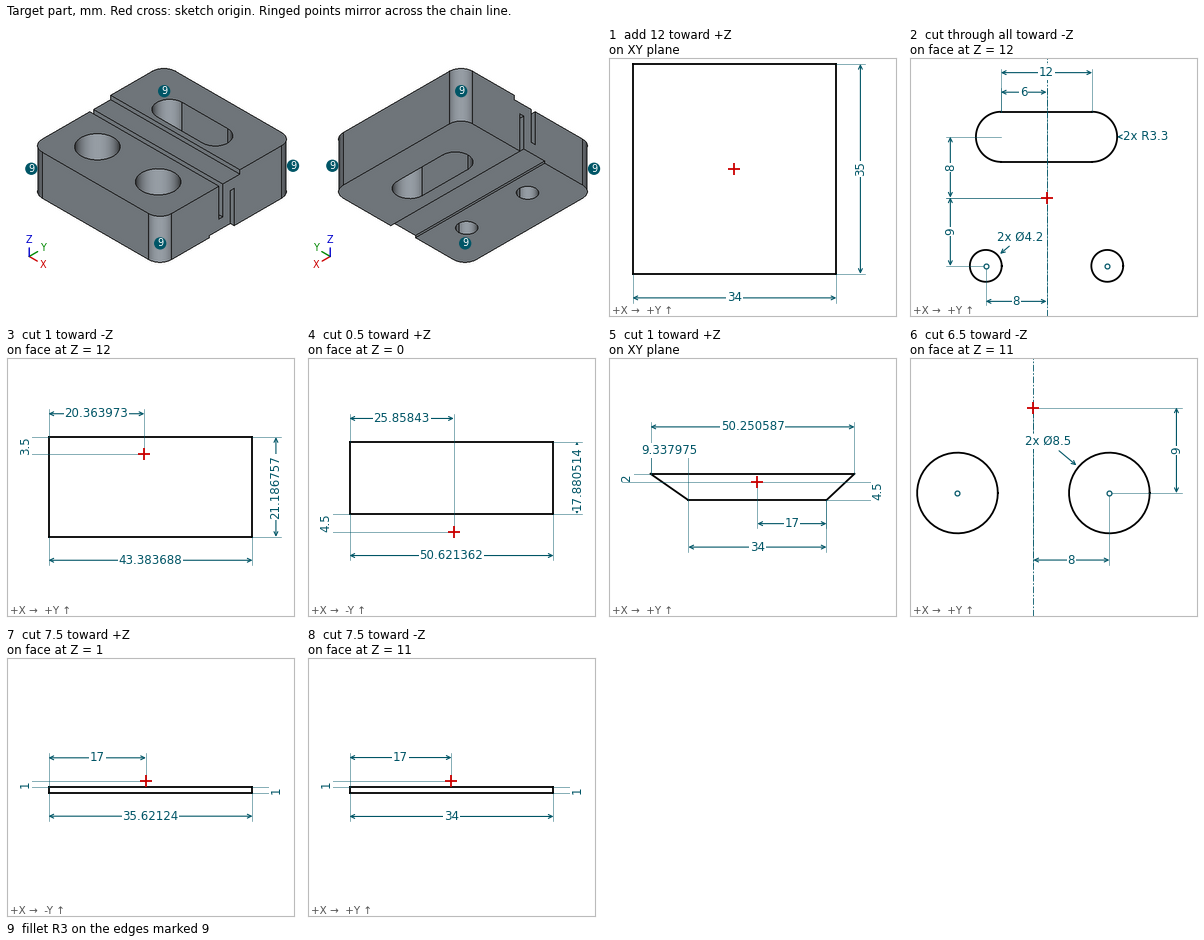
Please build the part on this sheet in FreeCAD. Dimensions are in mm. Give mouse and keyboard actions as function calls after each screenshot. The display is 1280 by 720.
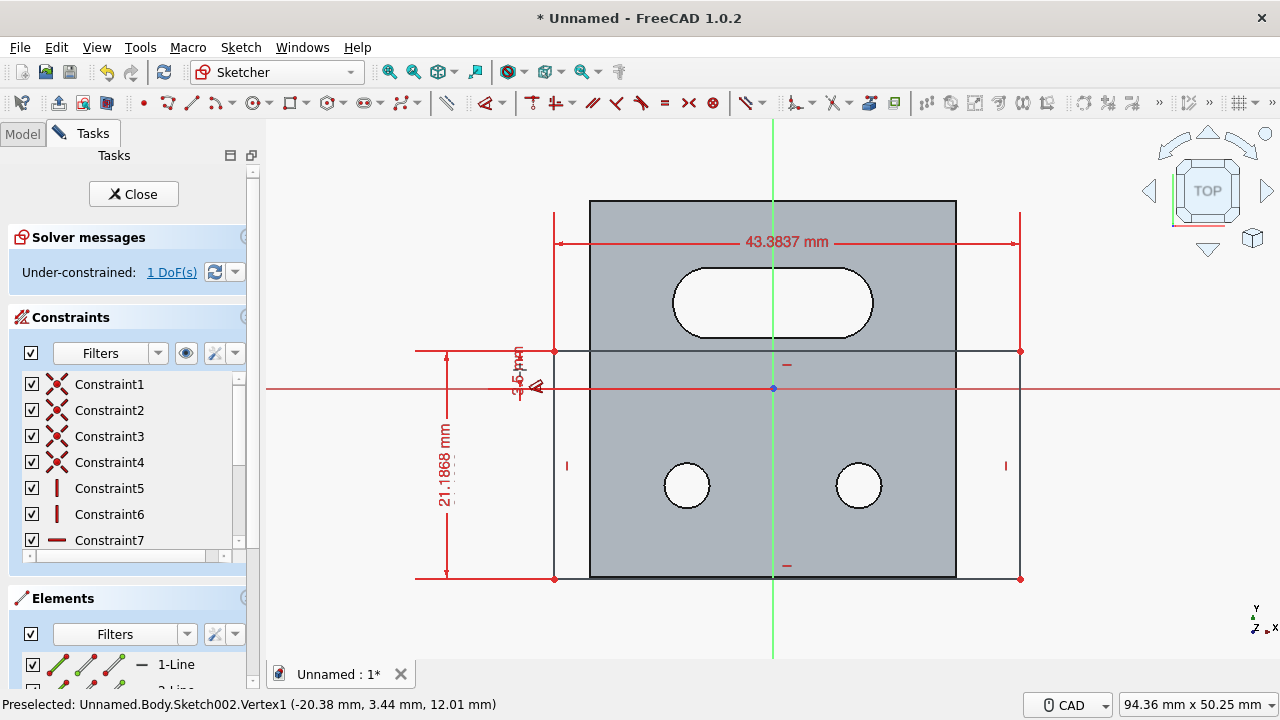
click(554, 351)
click(664, 317)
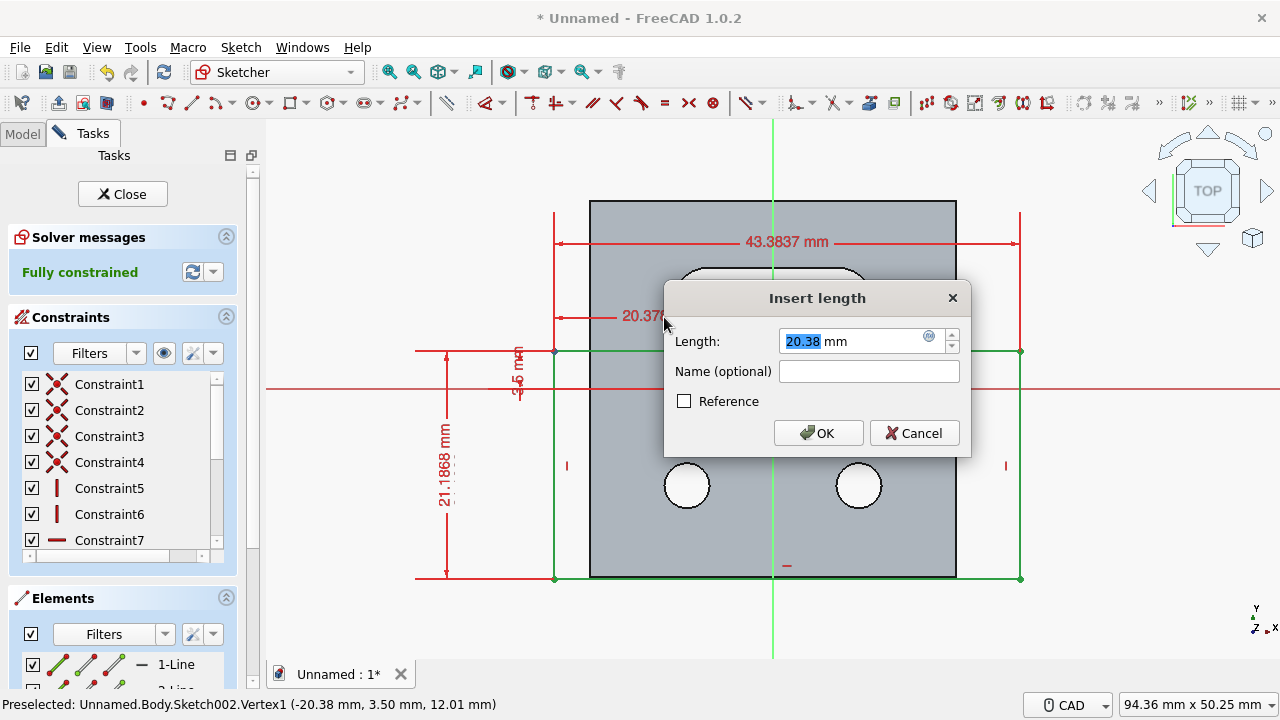
text(20.363973)
key(Return)
key(Escape)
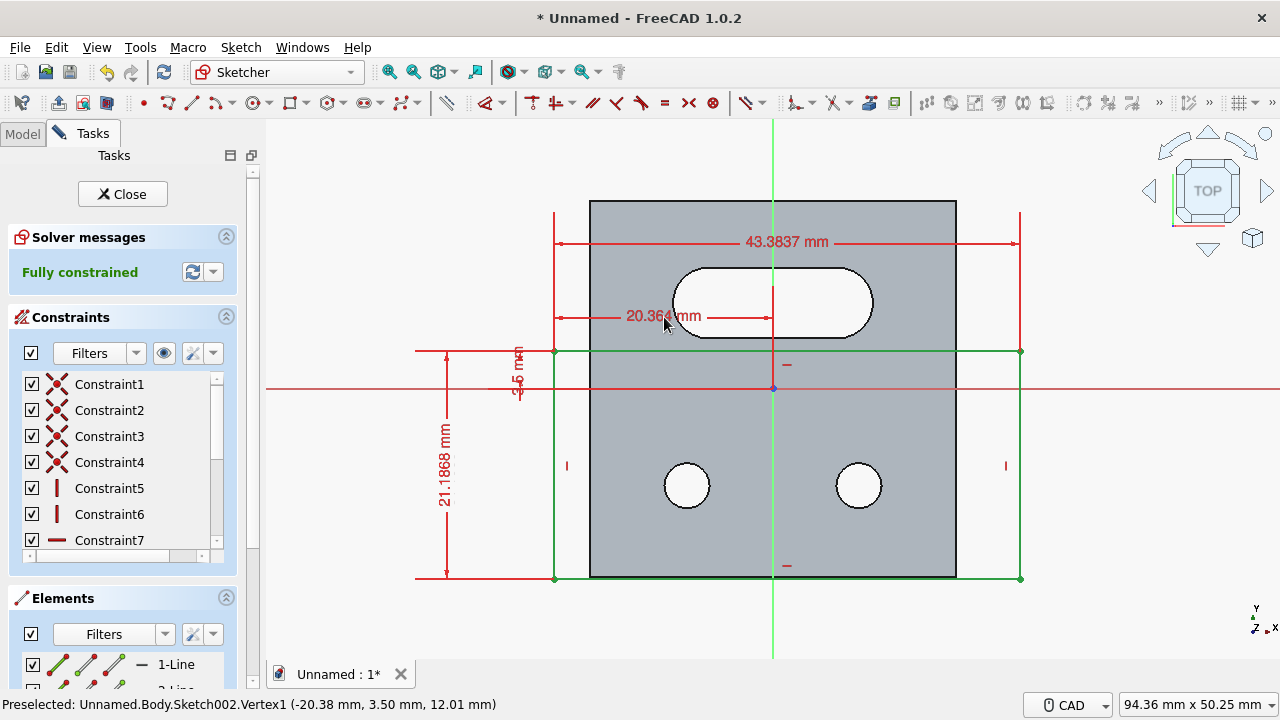
click(123, 194)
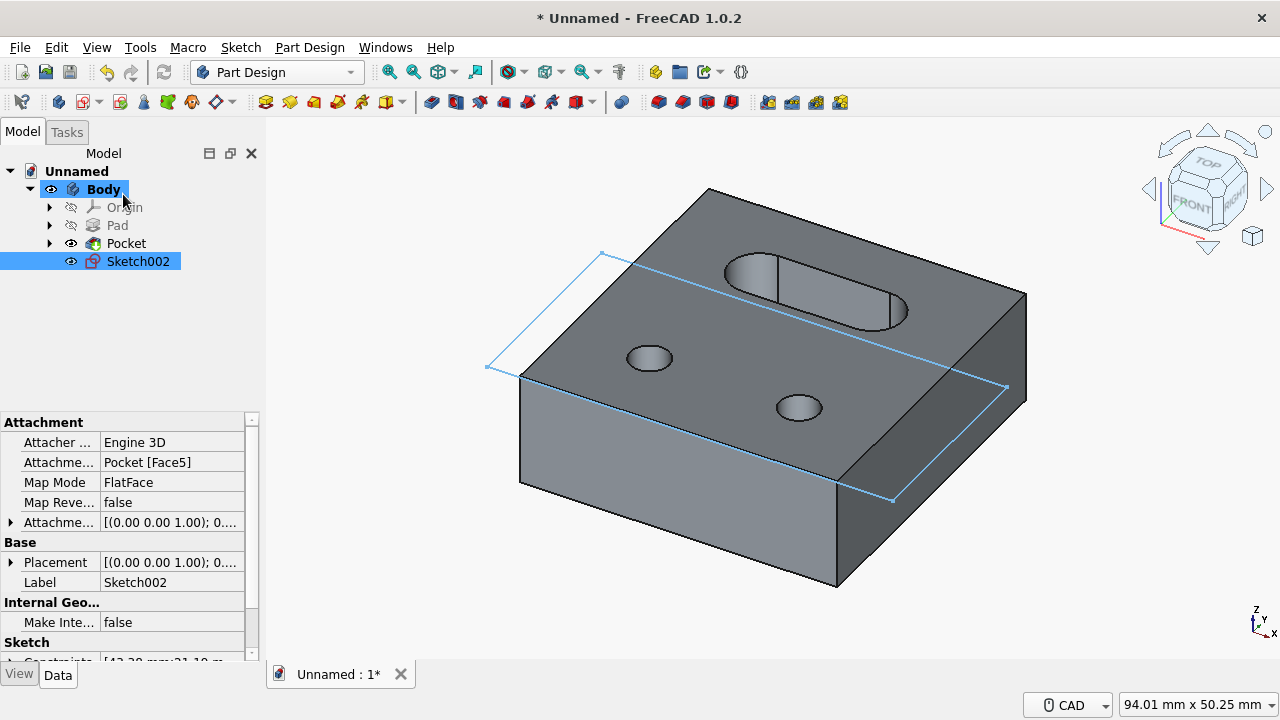
click(432, 102)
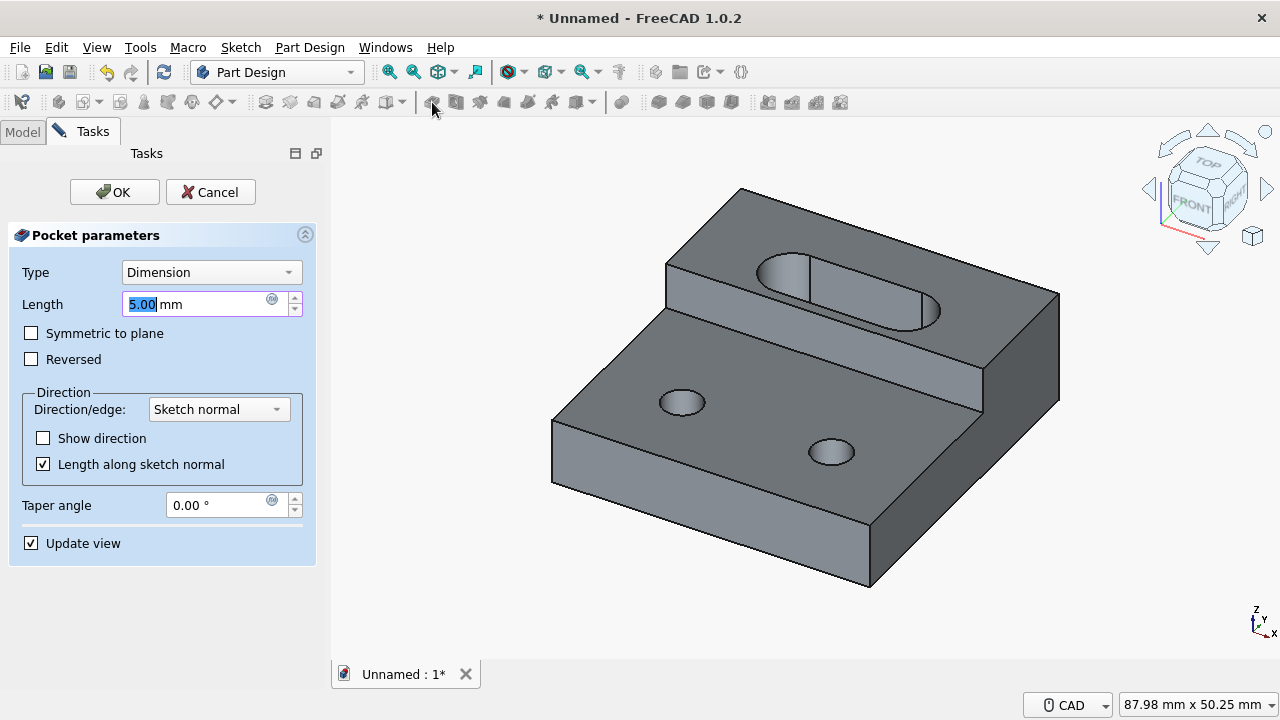
text(1)
key(Tab)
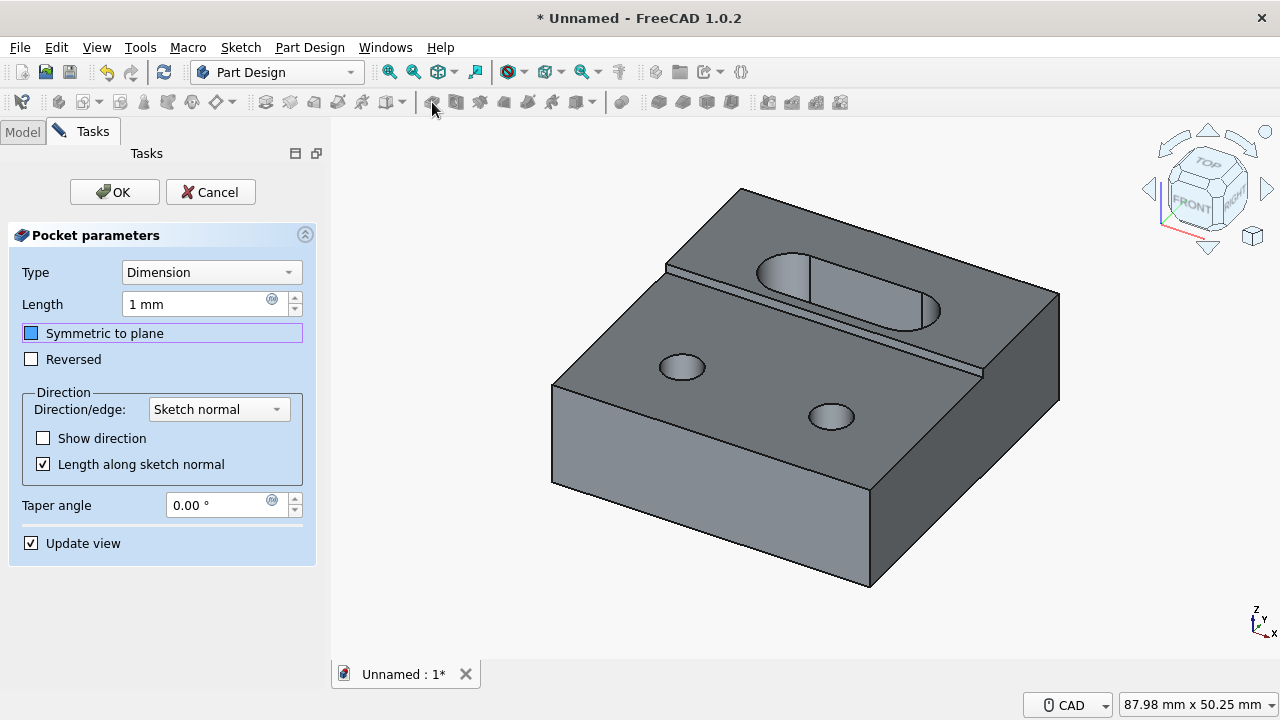
click(115, 192)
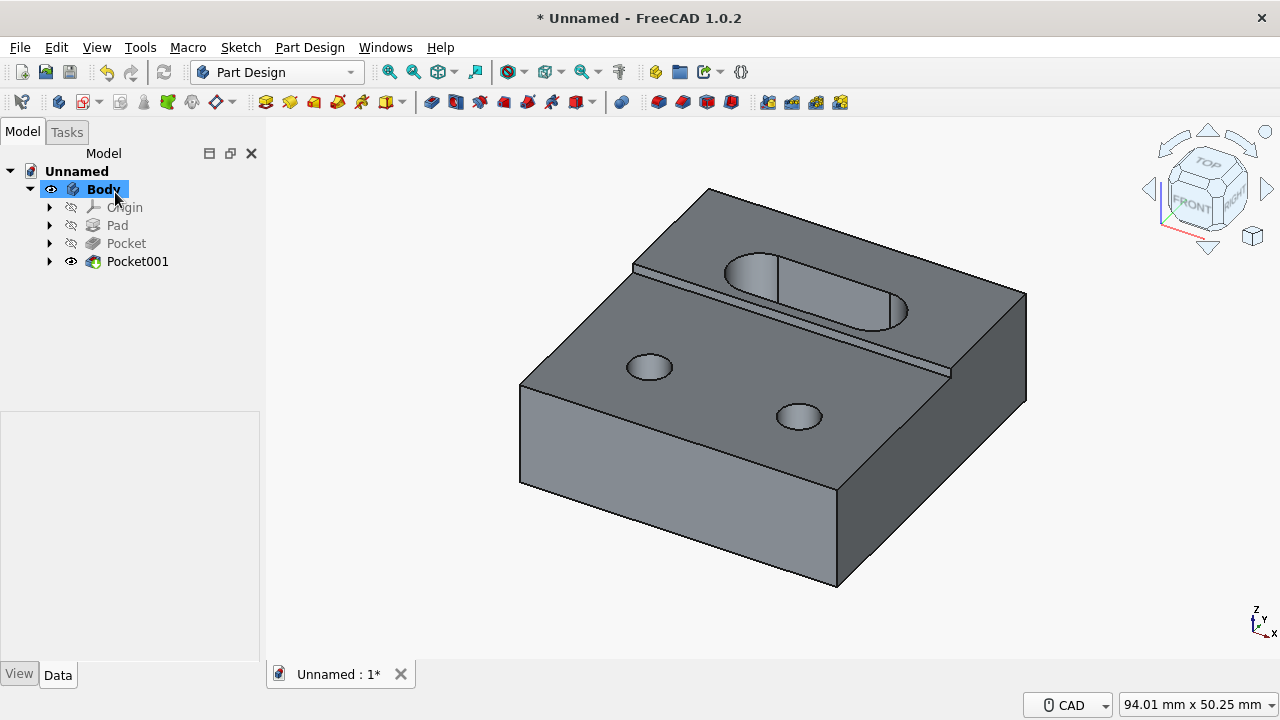
key(5)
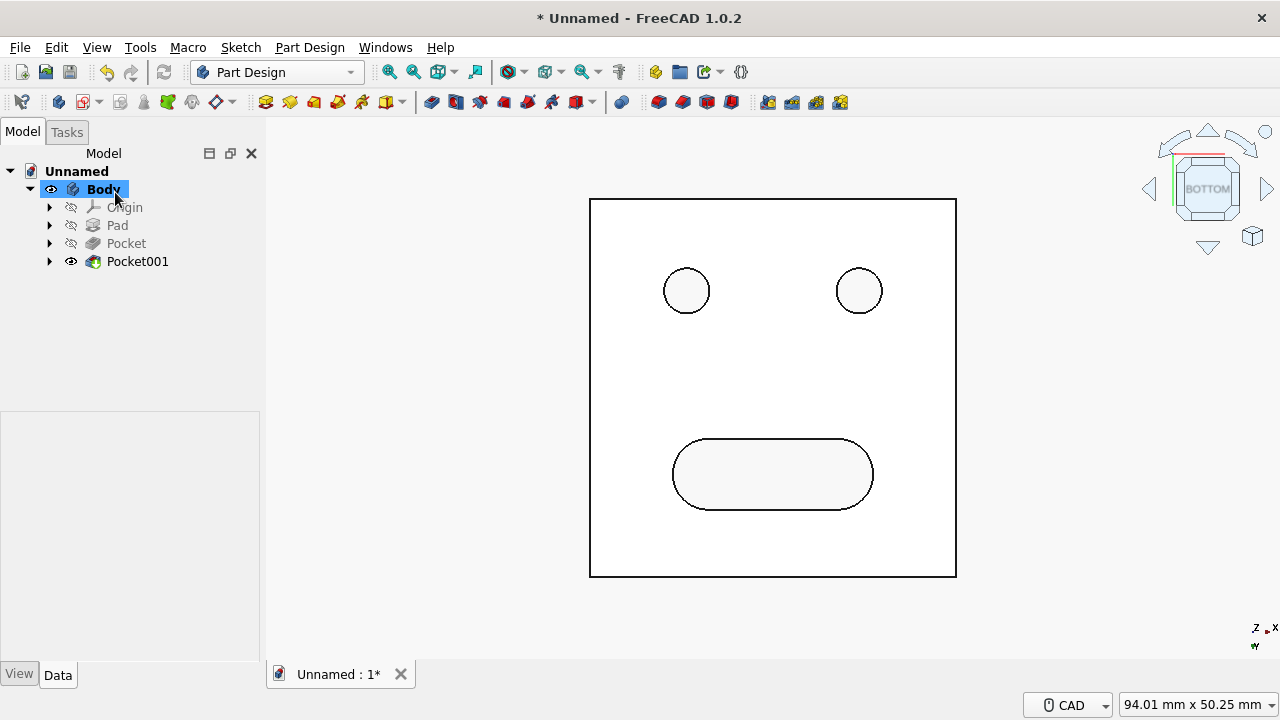
click(773, 333)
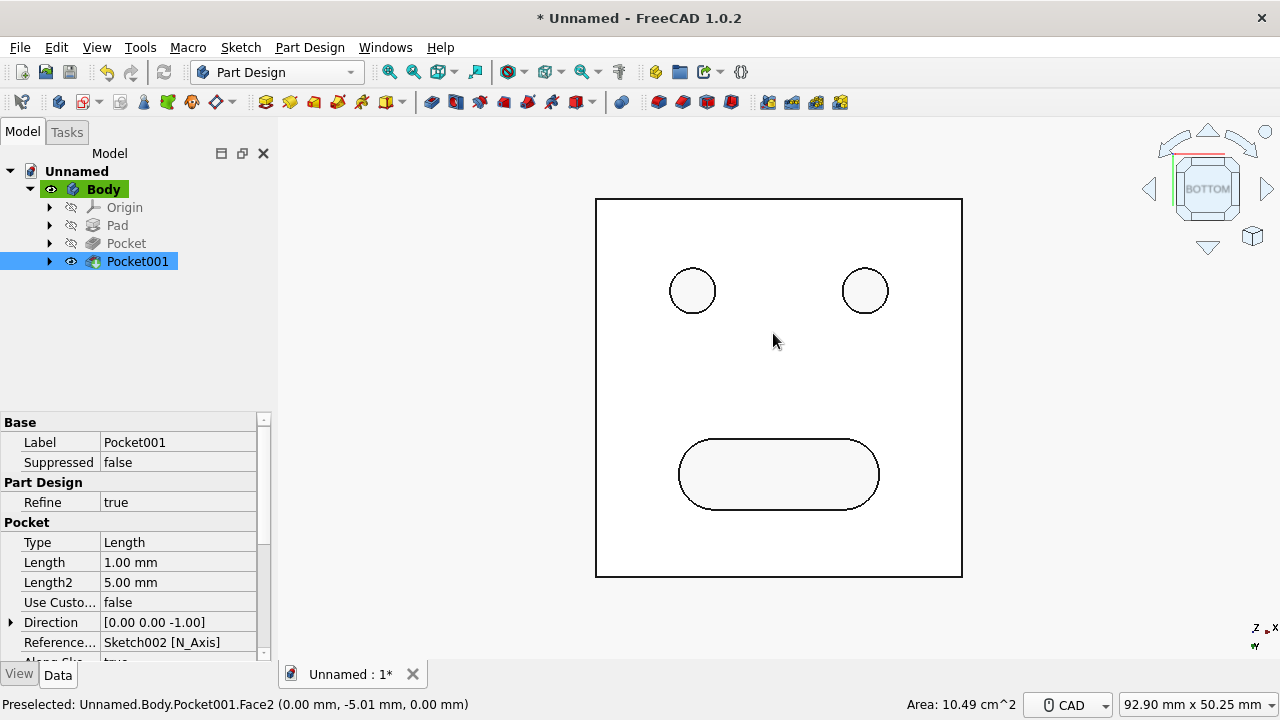
click(84, 102)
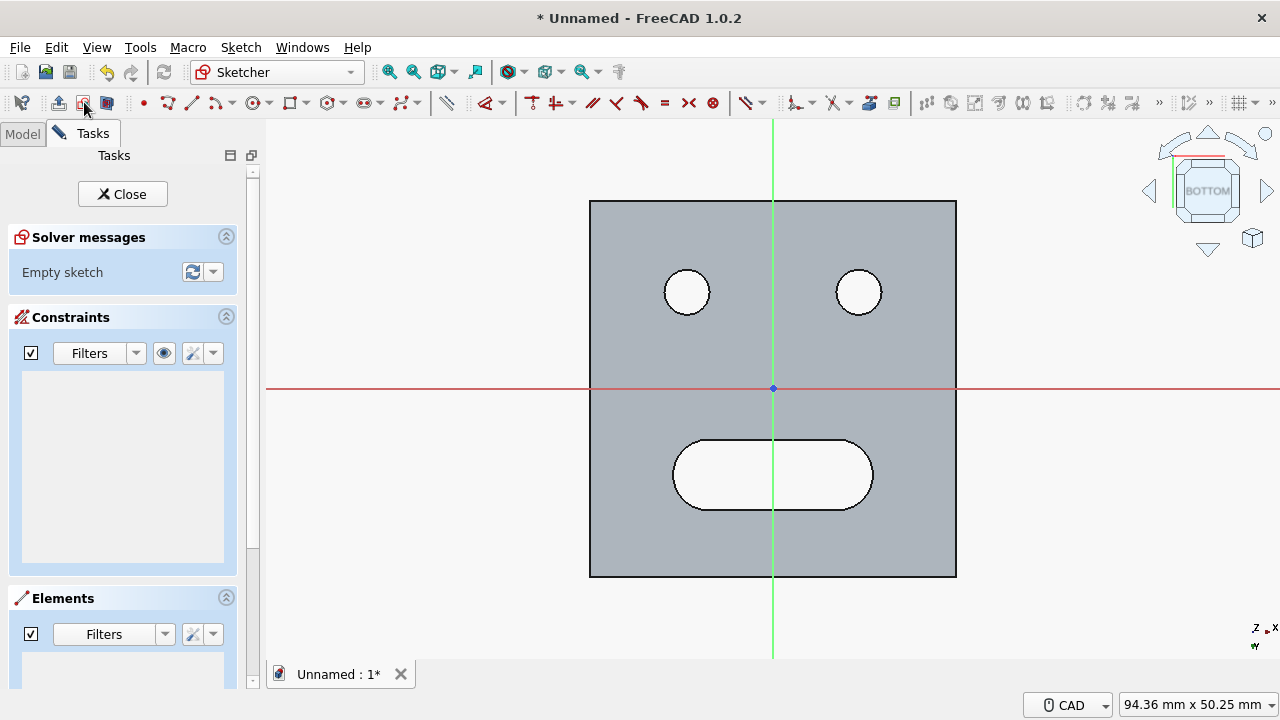
scroll(422, 631, down, 1)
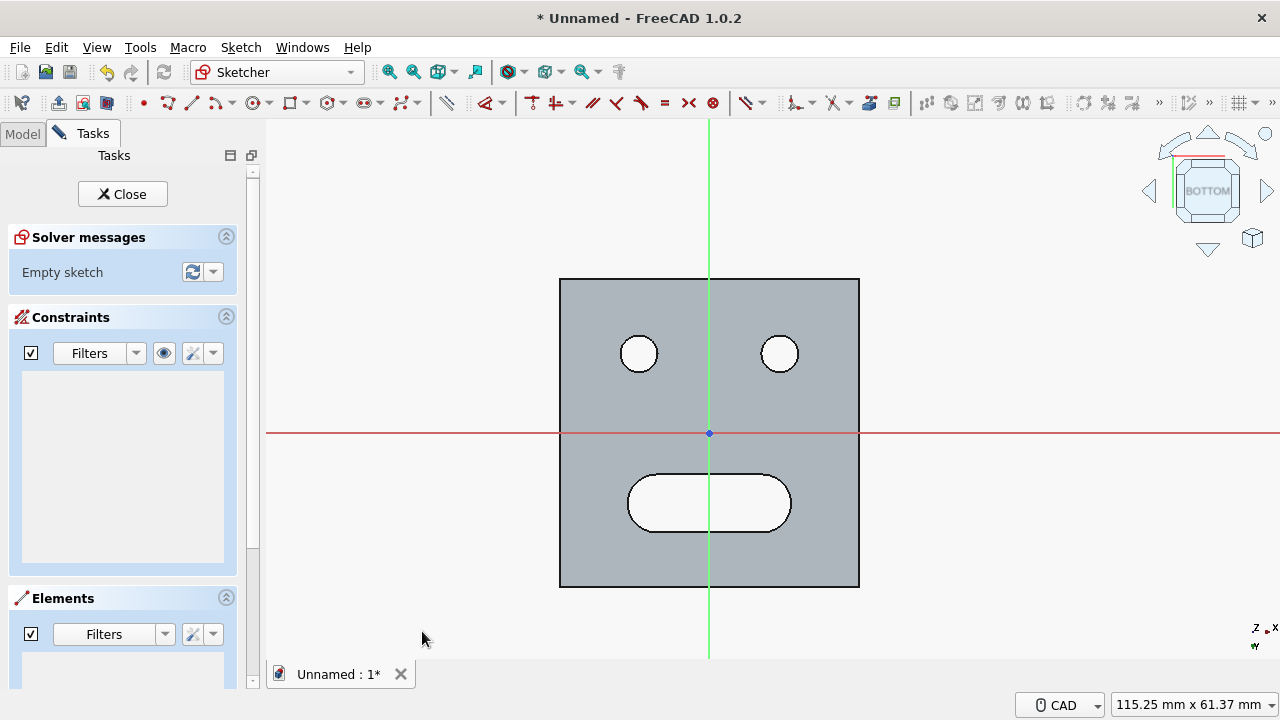
key(g)
key(r)